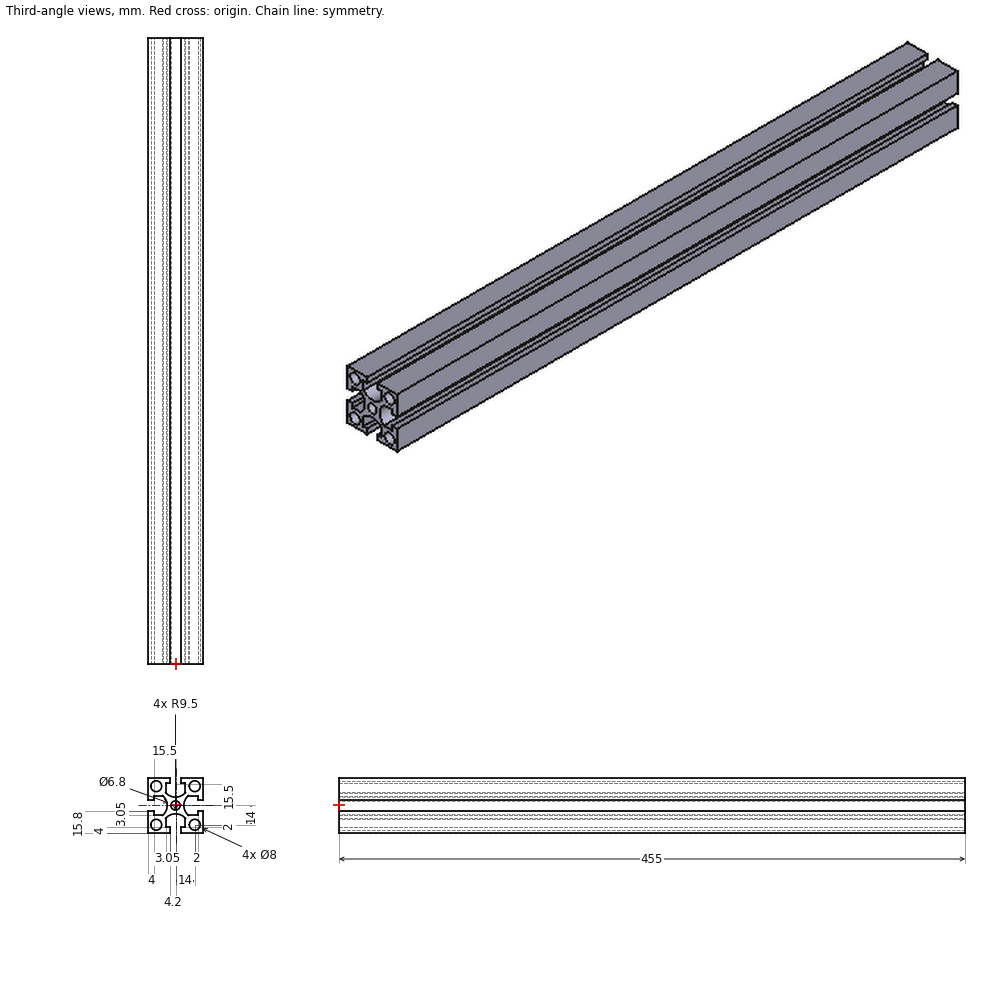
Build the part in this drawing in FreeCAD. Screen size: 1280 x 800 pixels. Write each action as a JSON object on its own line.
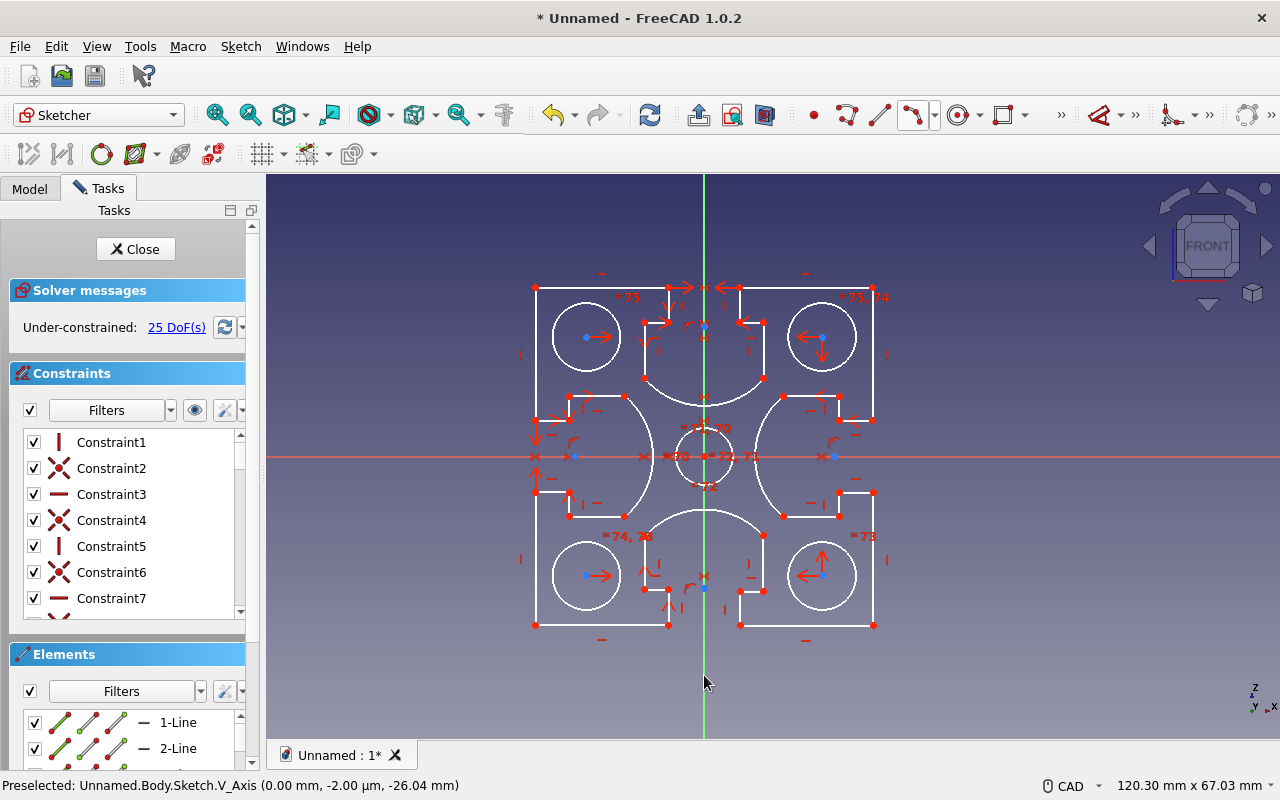
{"action": "left_click", "coordinate": [625, 517]}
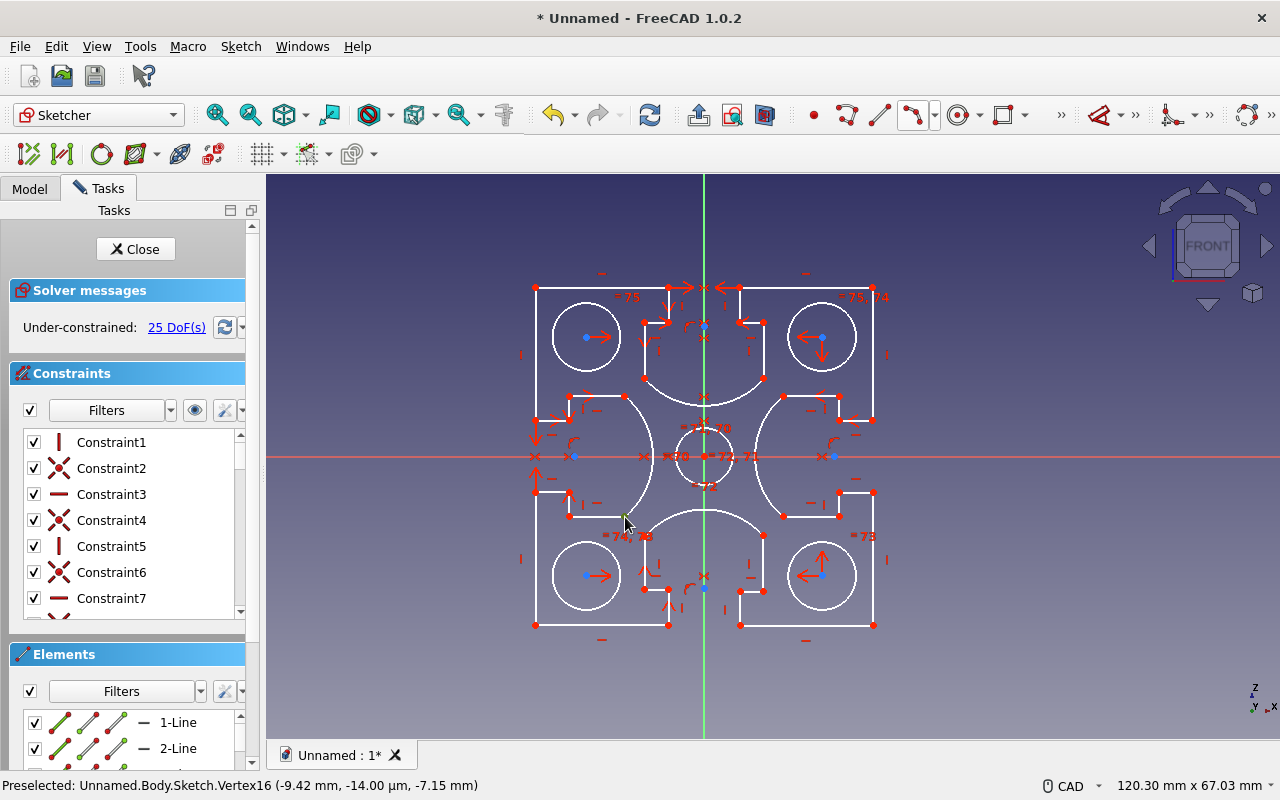
{"action": "left_click", "coordinate": [783, 517]}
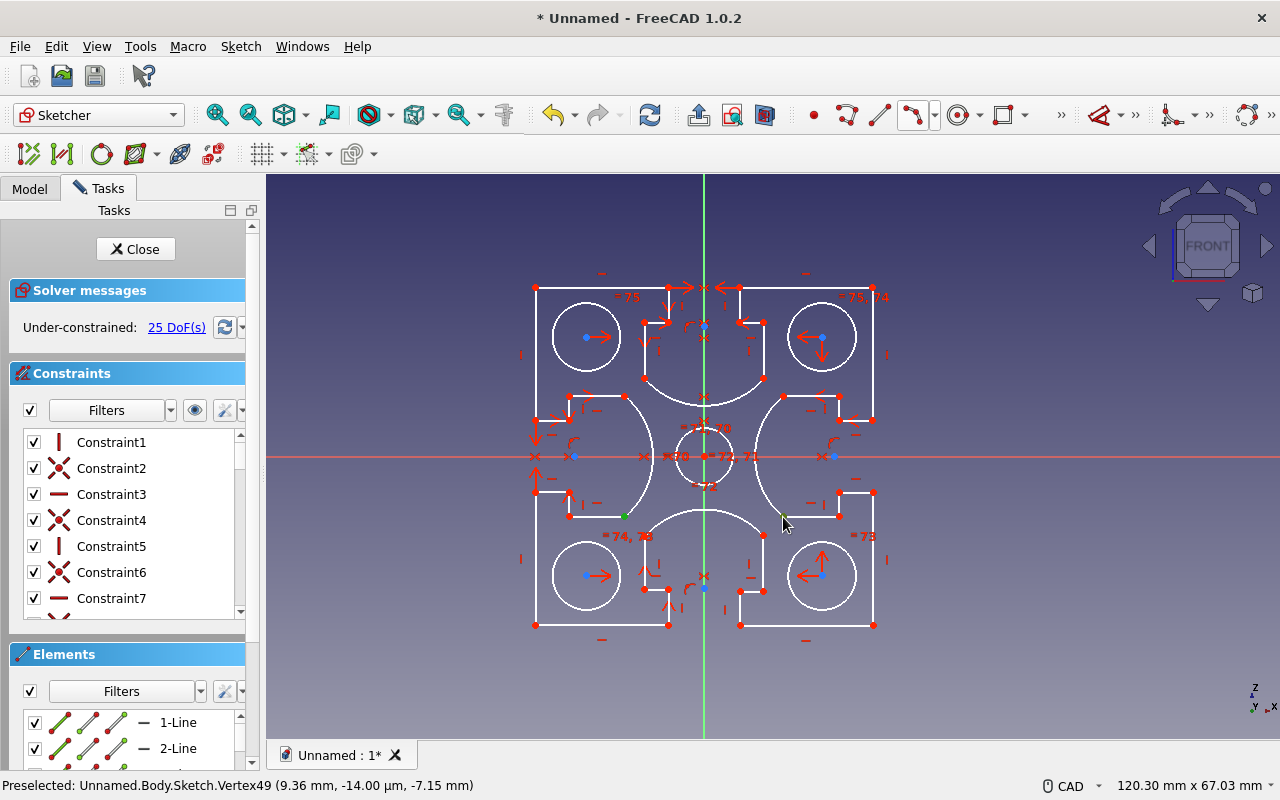
{"action": "left_click", "coordinate": [704, 675]}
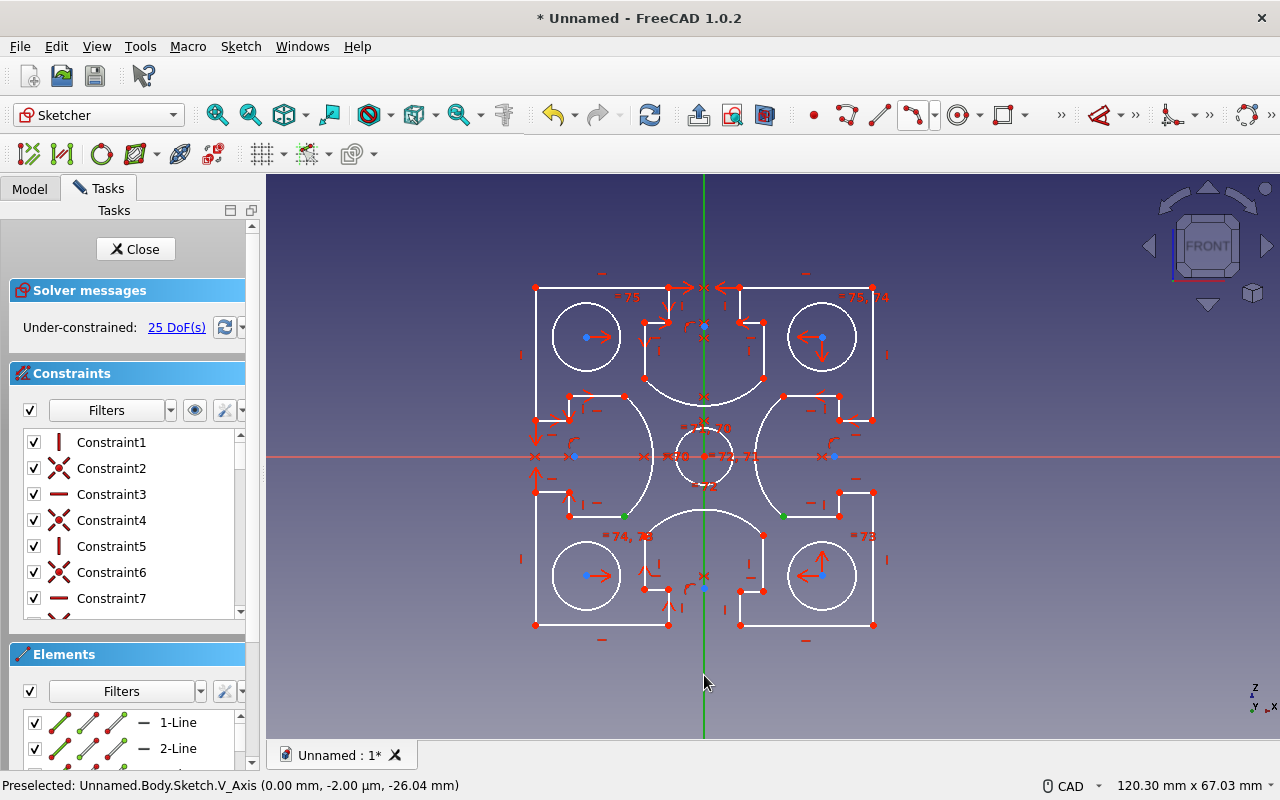
{"action": "key", "text": "s"}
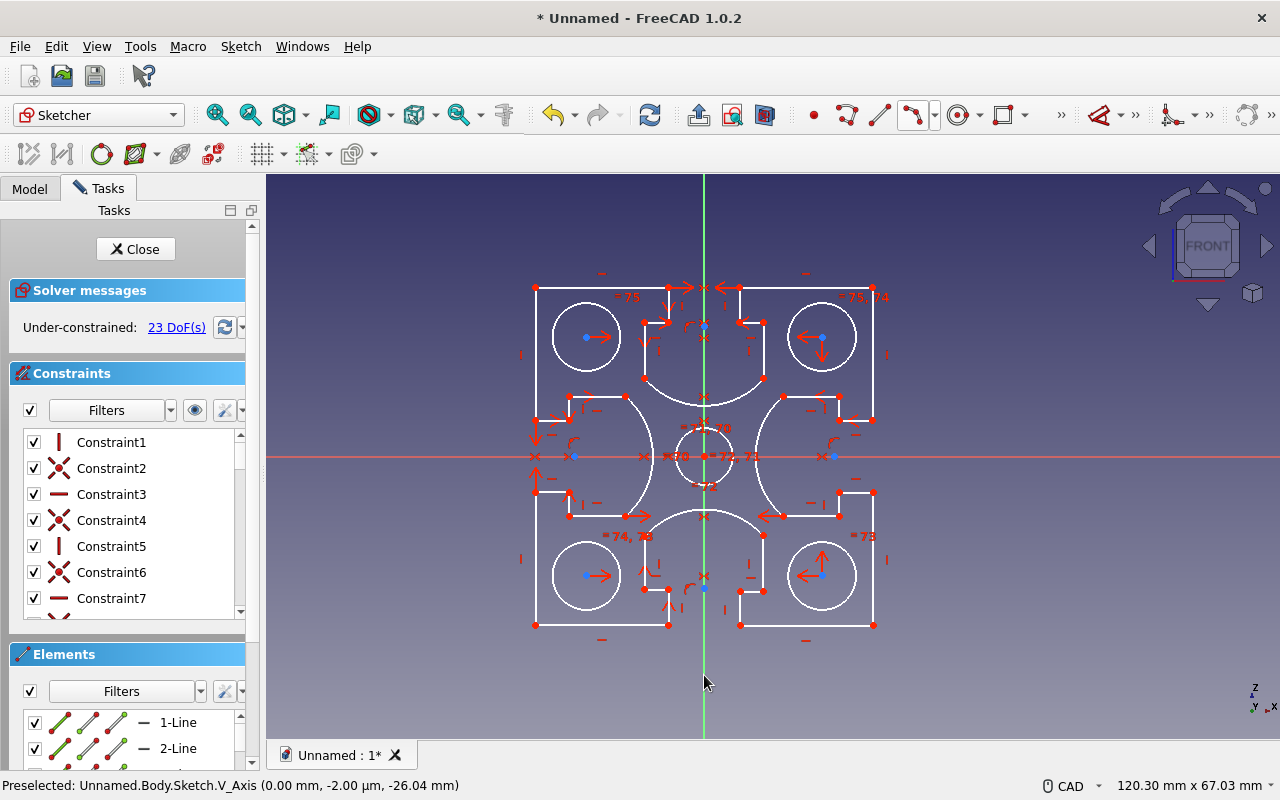
{"action": "left_click", "coordinate": [569, 492]}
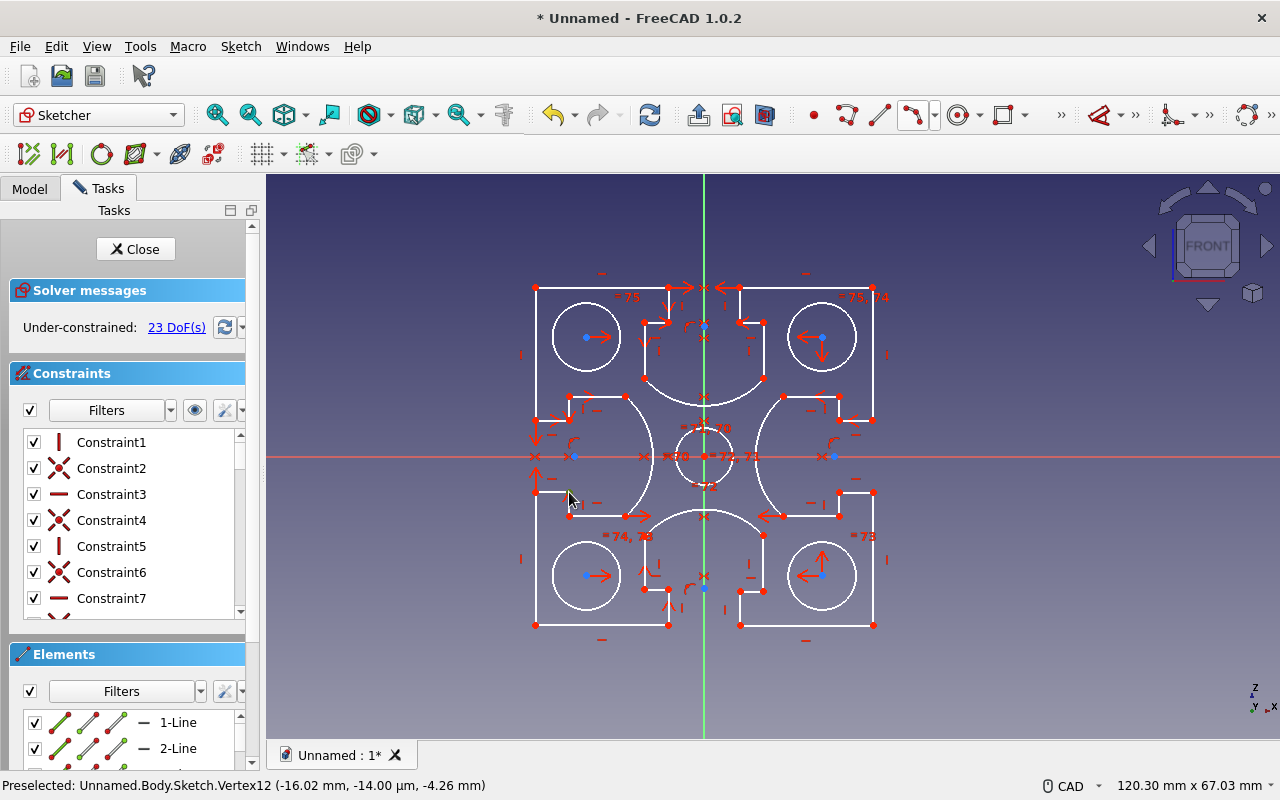
{"action": "left_click", "coordinate": [839, 493]}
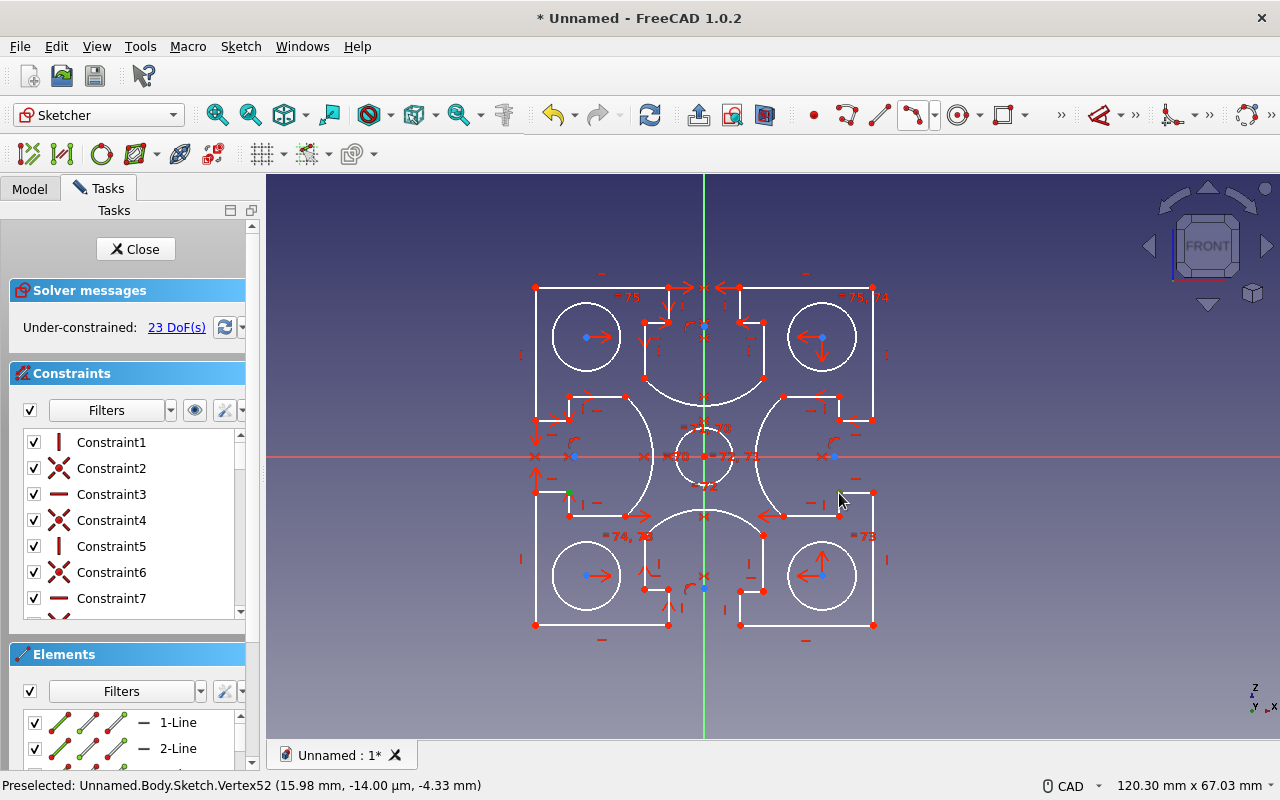
{"action": "left_click", "coordinate": [704, 675]}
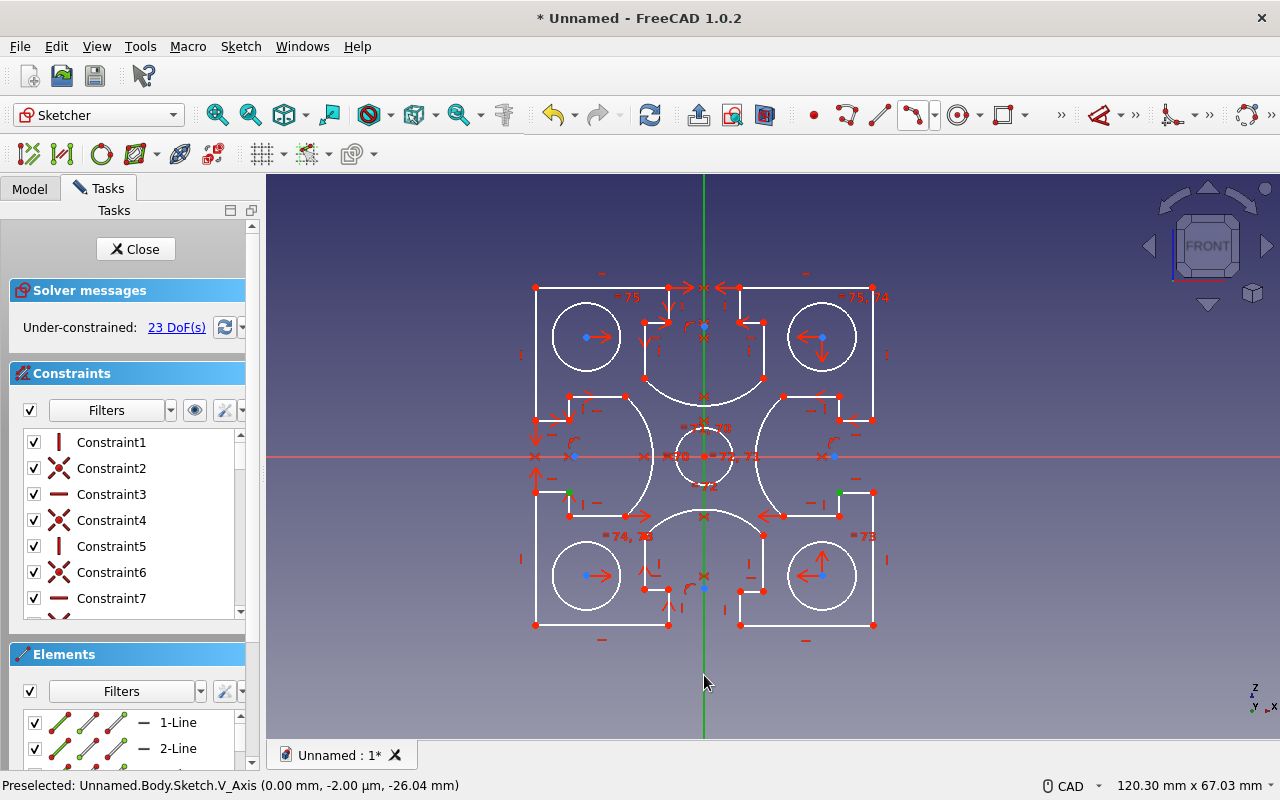
{"action": "key", "text": "s"}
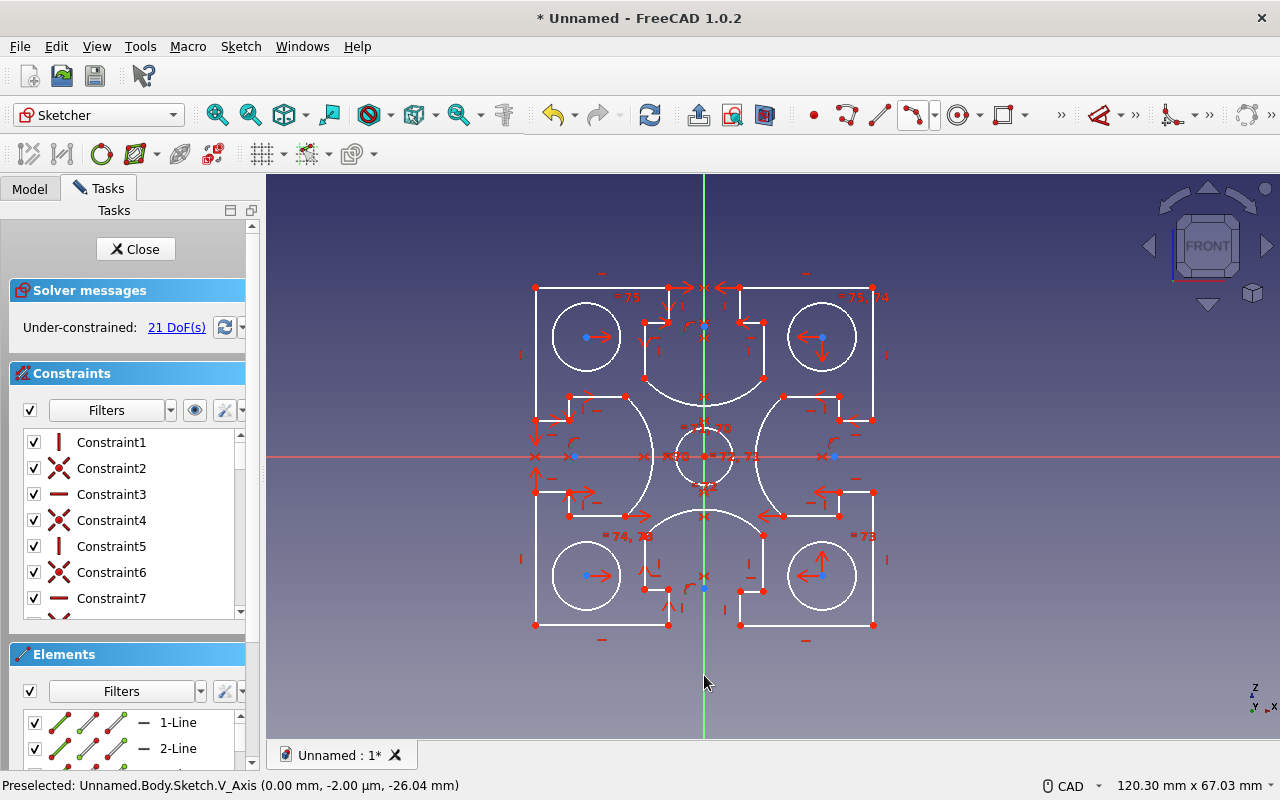
{"action": "left_click", "coordinate": [536, 625]}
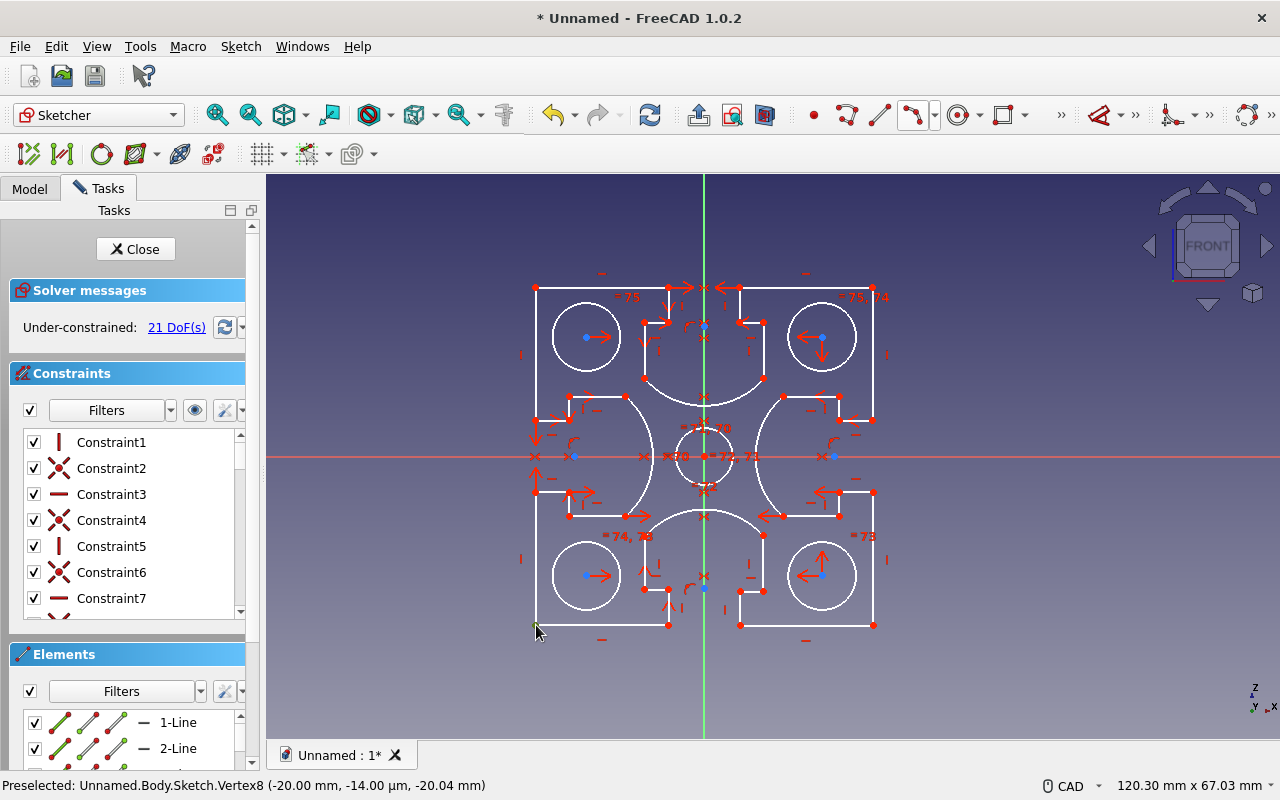
{"action": "left_click", "coordinate": [873, 626]}